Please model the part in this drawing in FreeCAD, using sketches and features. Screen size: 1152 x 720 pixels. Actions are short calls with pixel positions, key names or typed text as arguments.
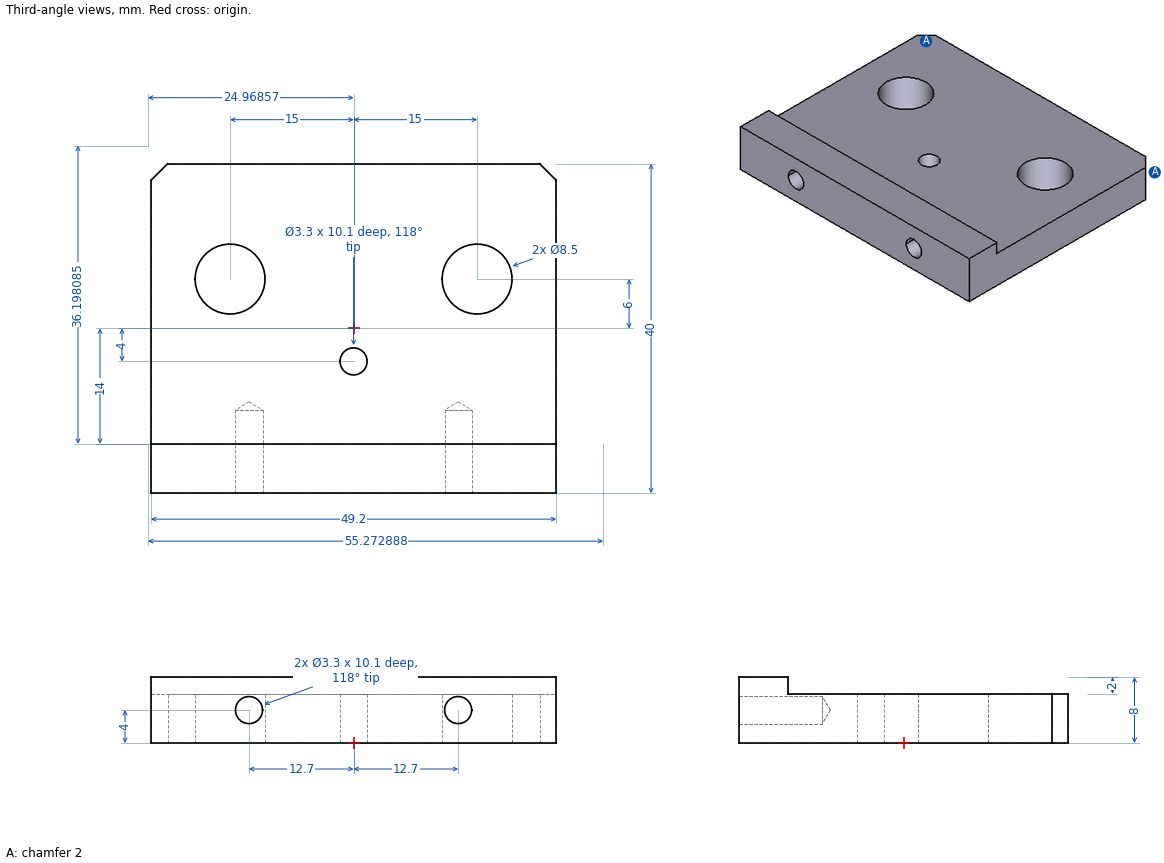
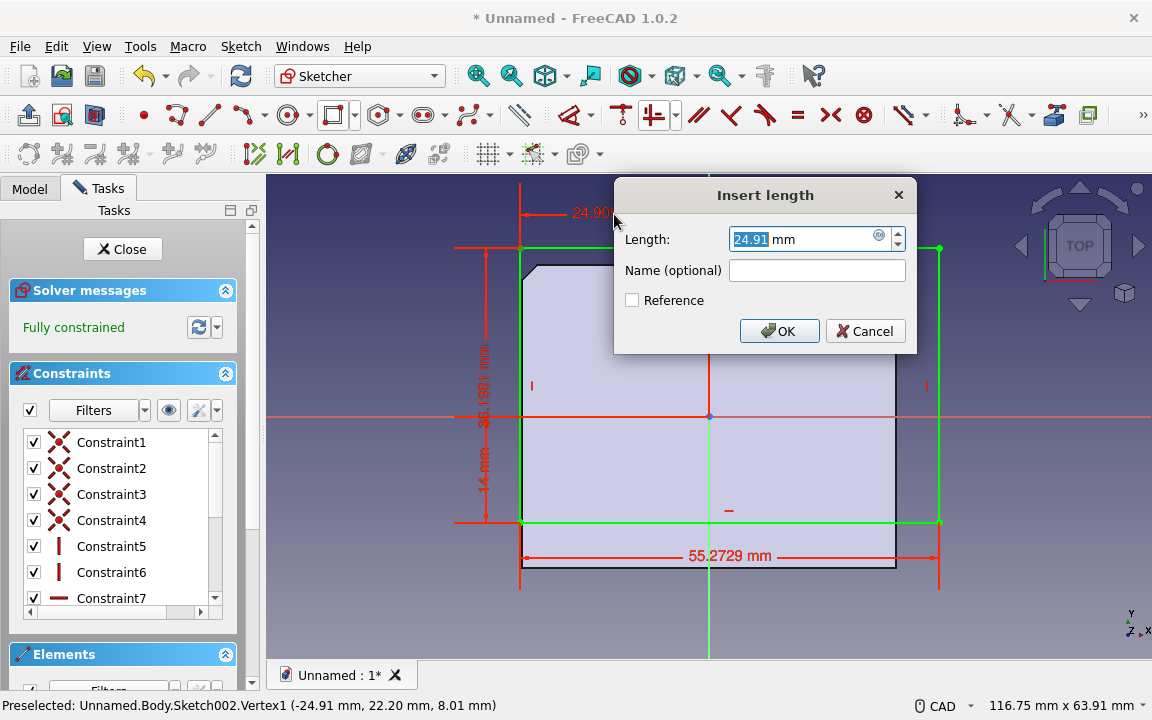
text(24.96857)
key(Return)
key(Escape)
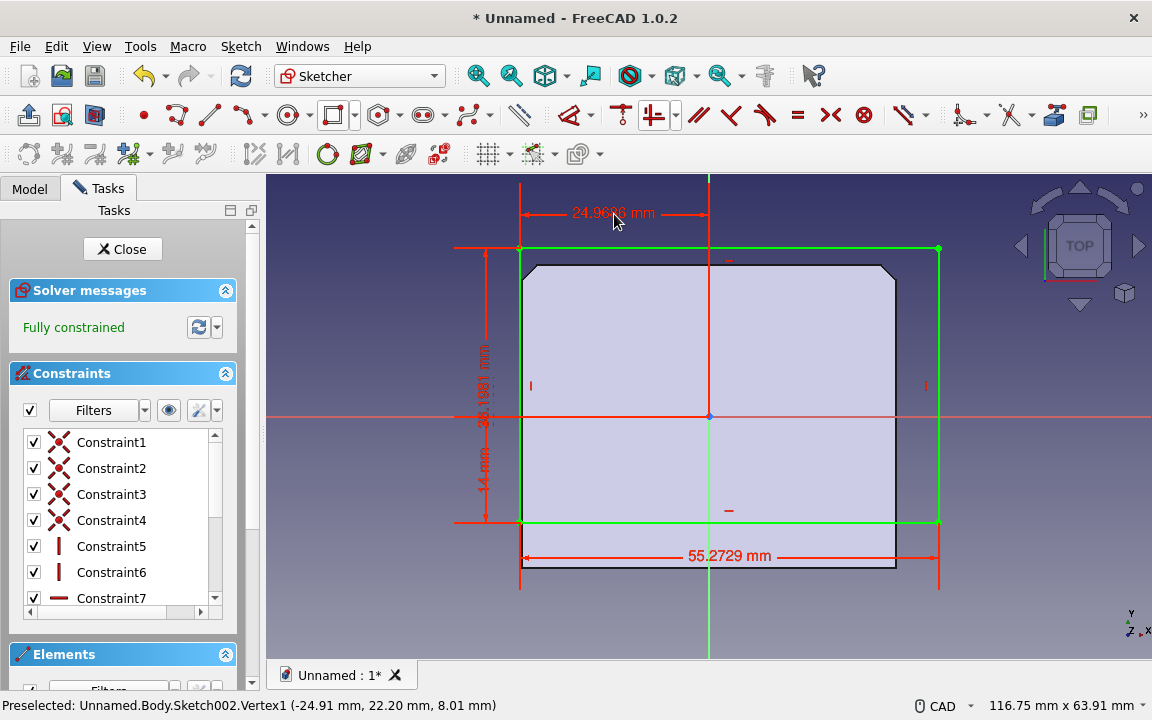
click(123, 249)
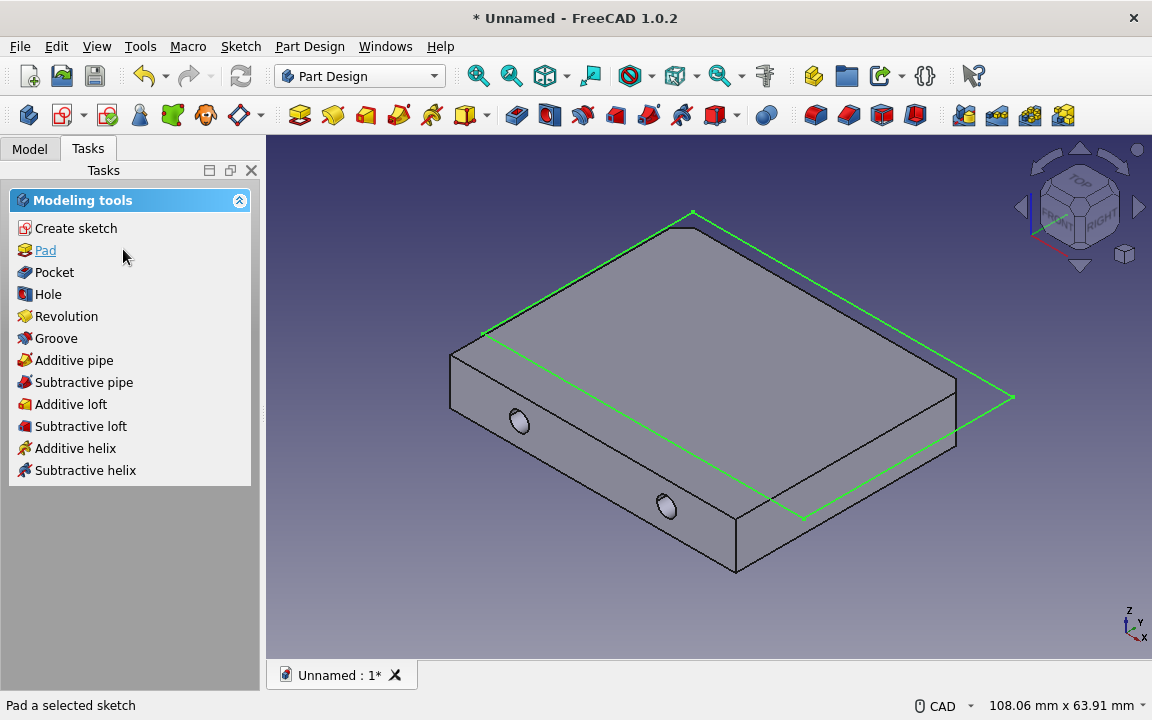
click(517, 116)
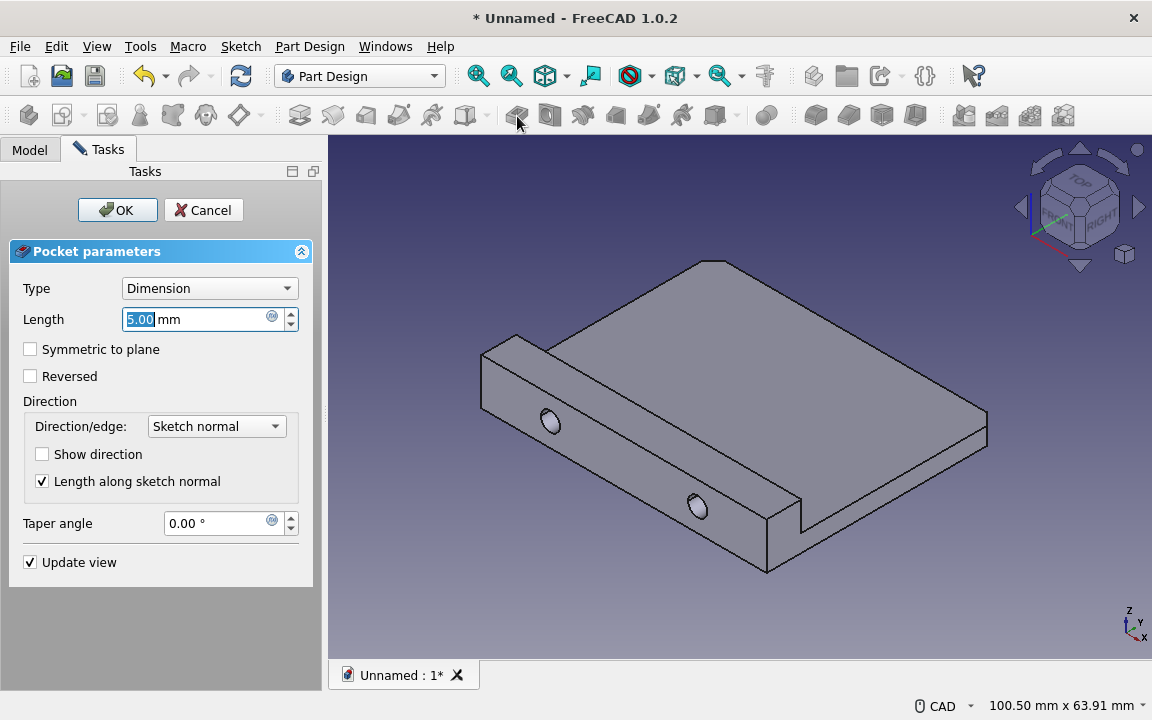
text(2)
key(Tab)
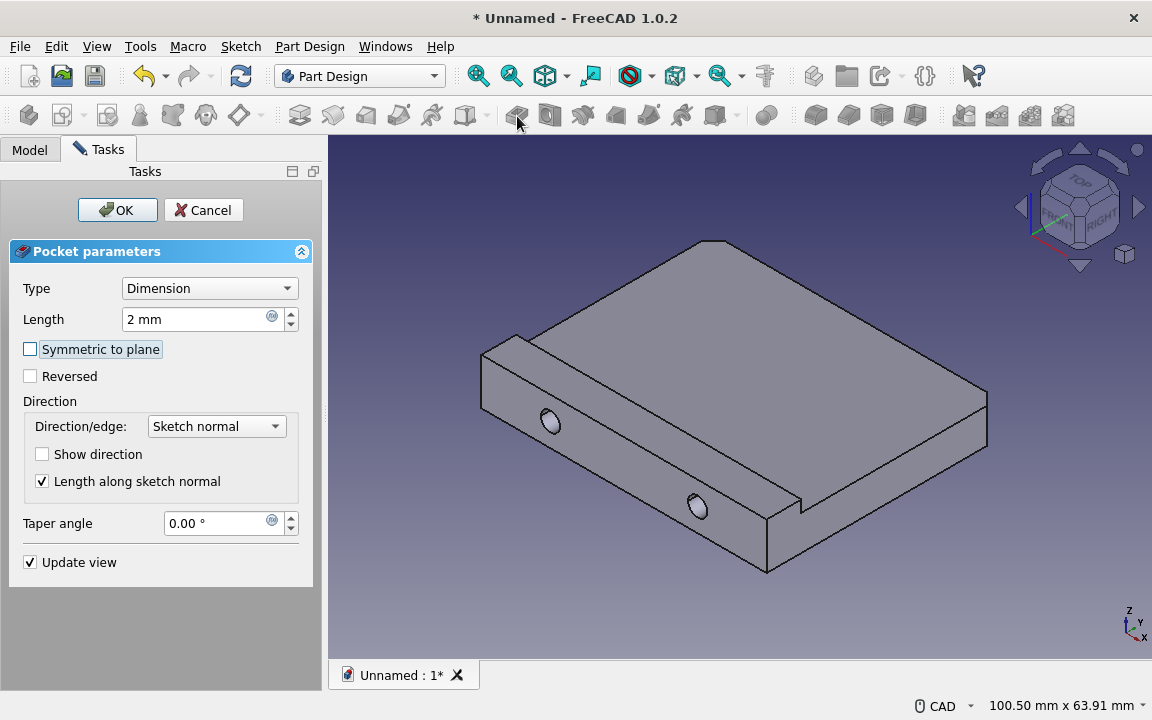
click(118, 210)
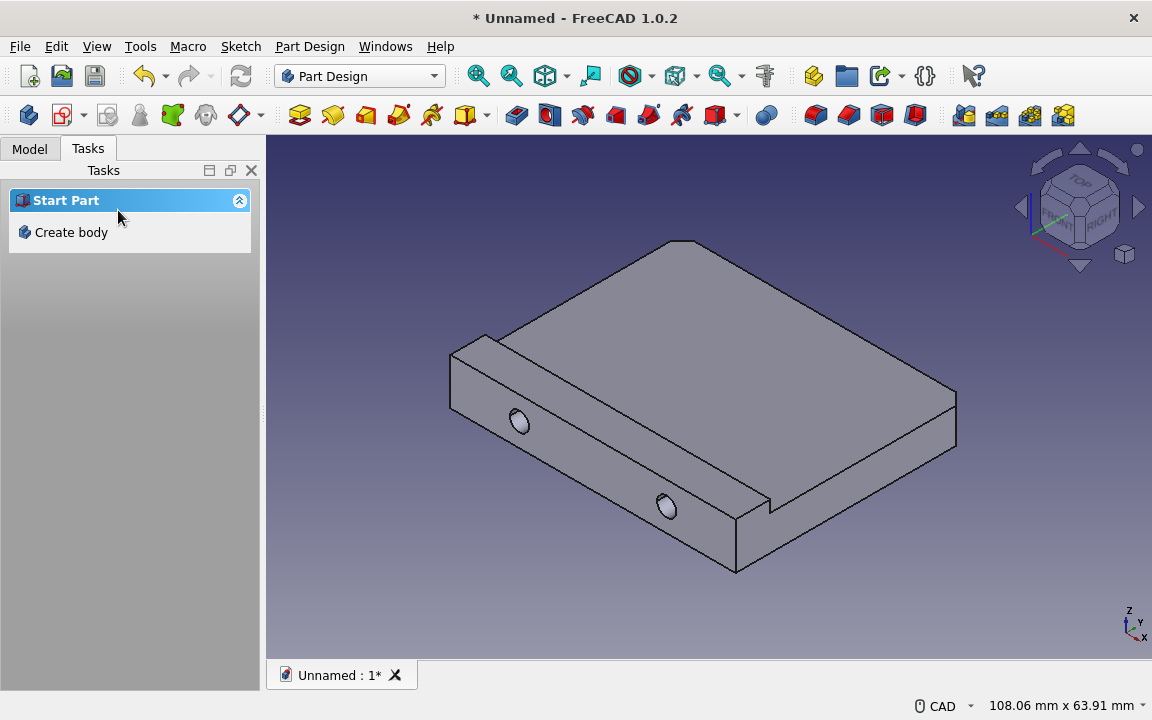
key(5)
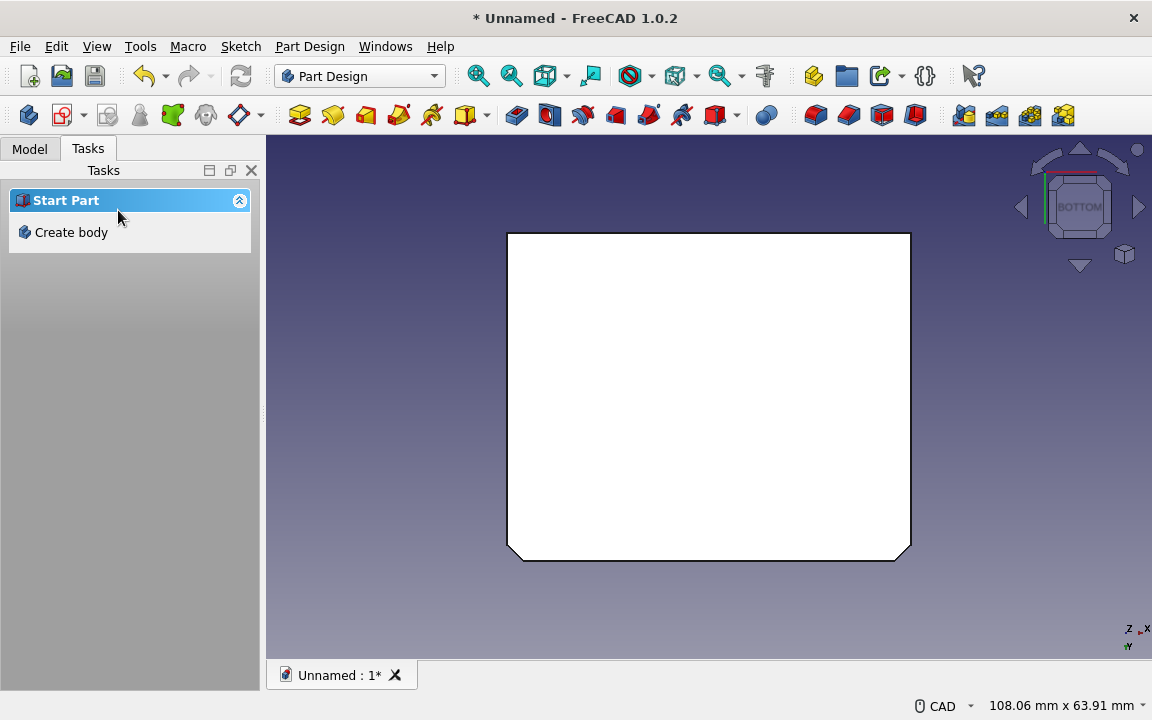
click(709, 396)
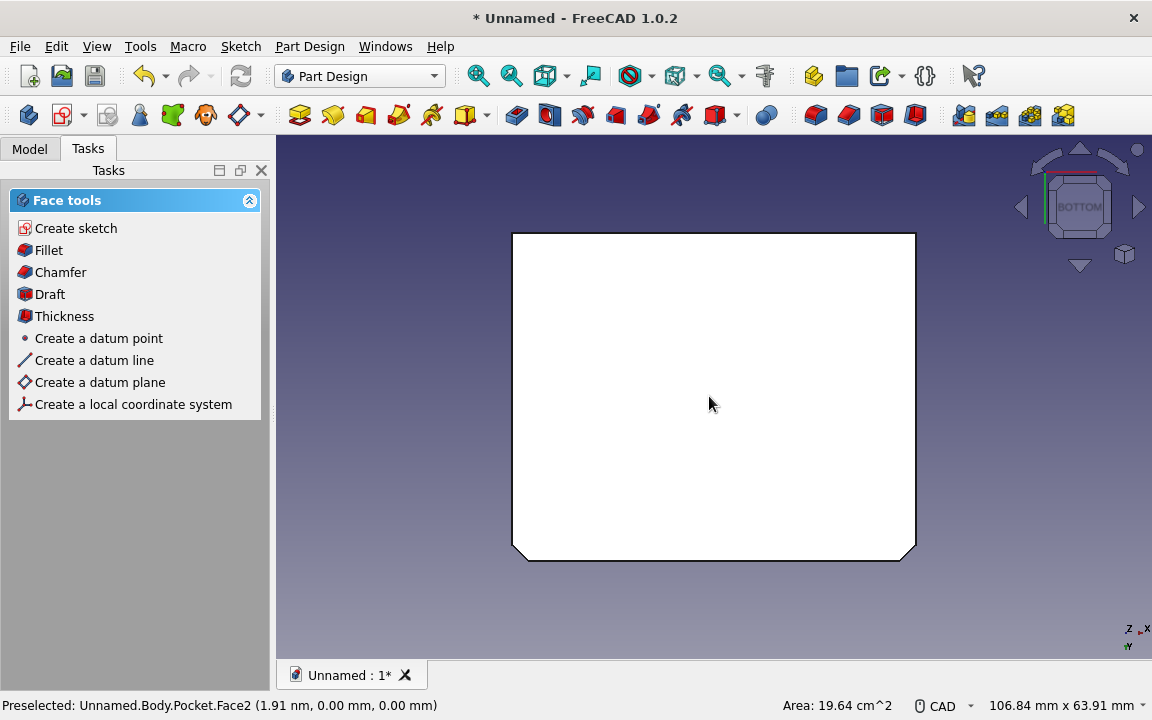
click(62, 116)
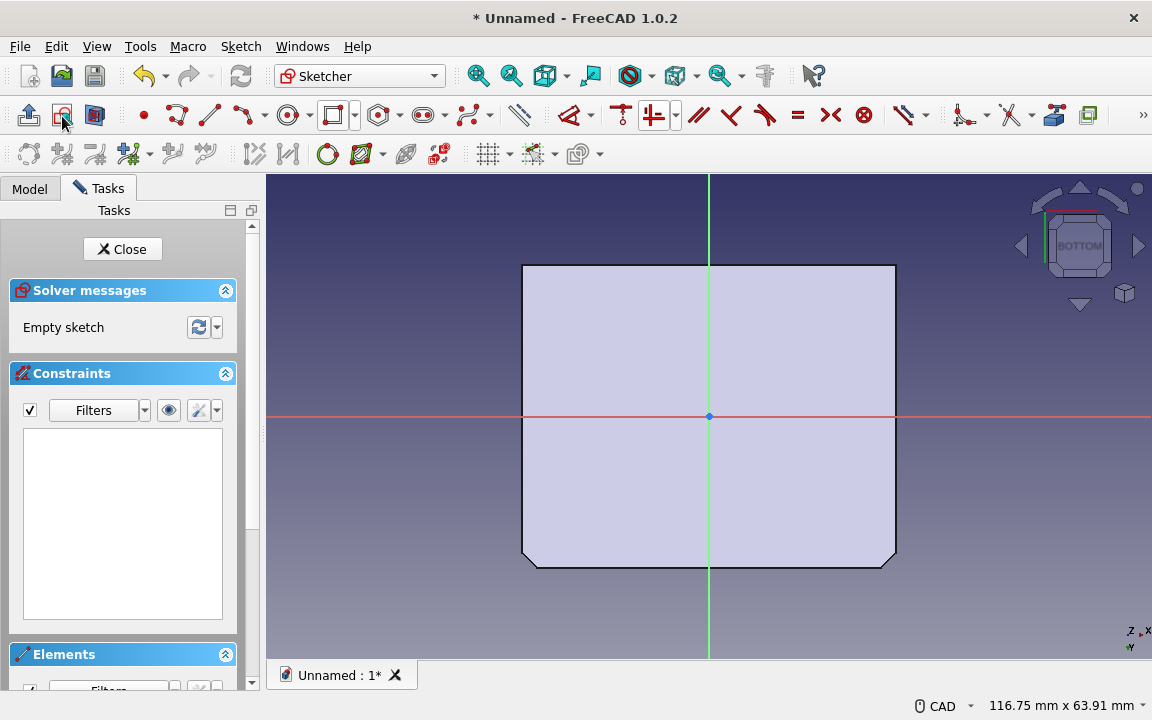
scroll(792, 503, up, 3)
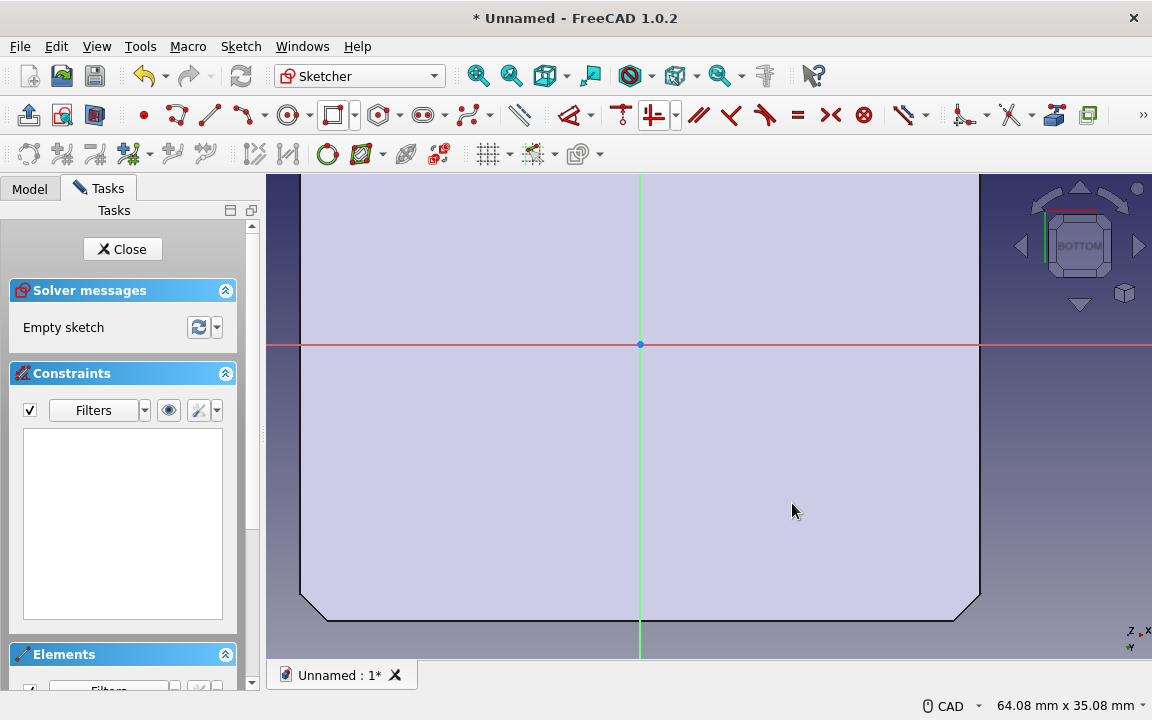
click(288, 116)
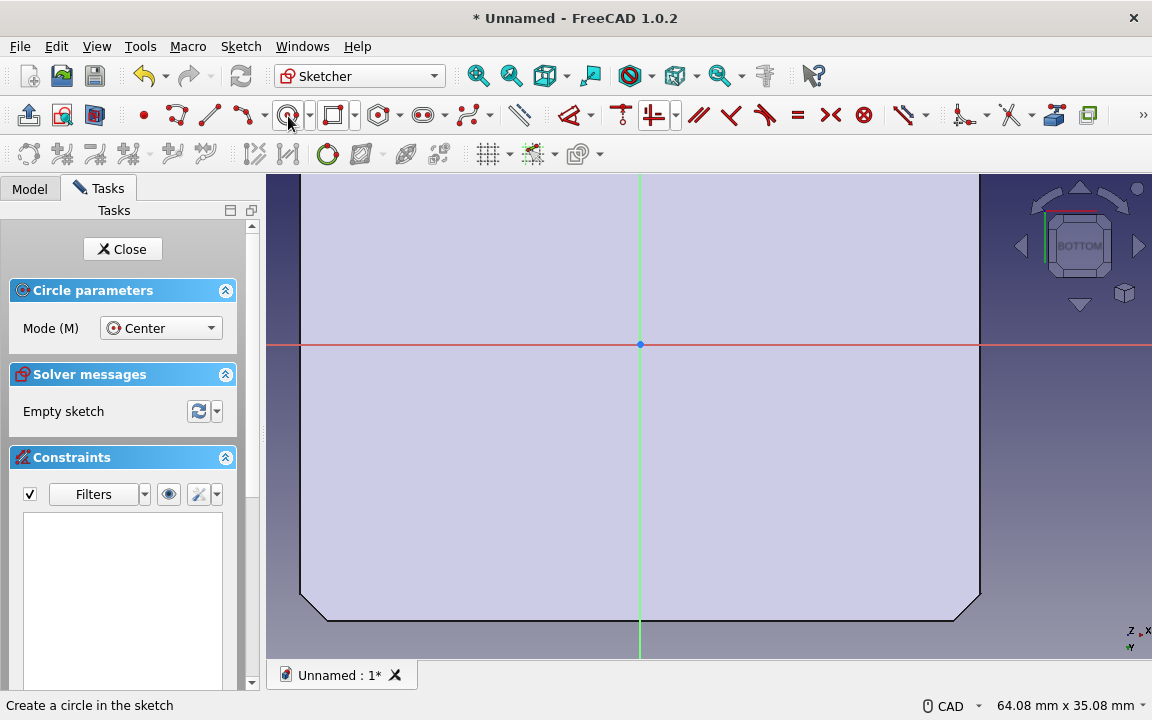
click(848, 428)
click(889, 386)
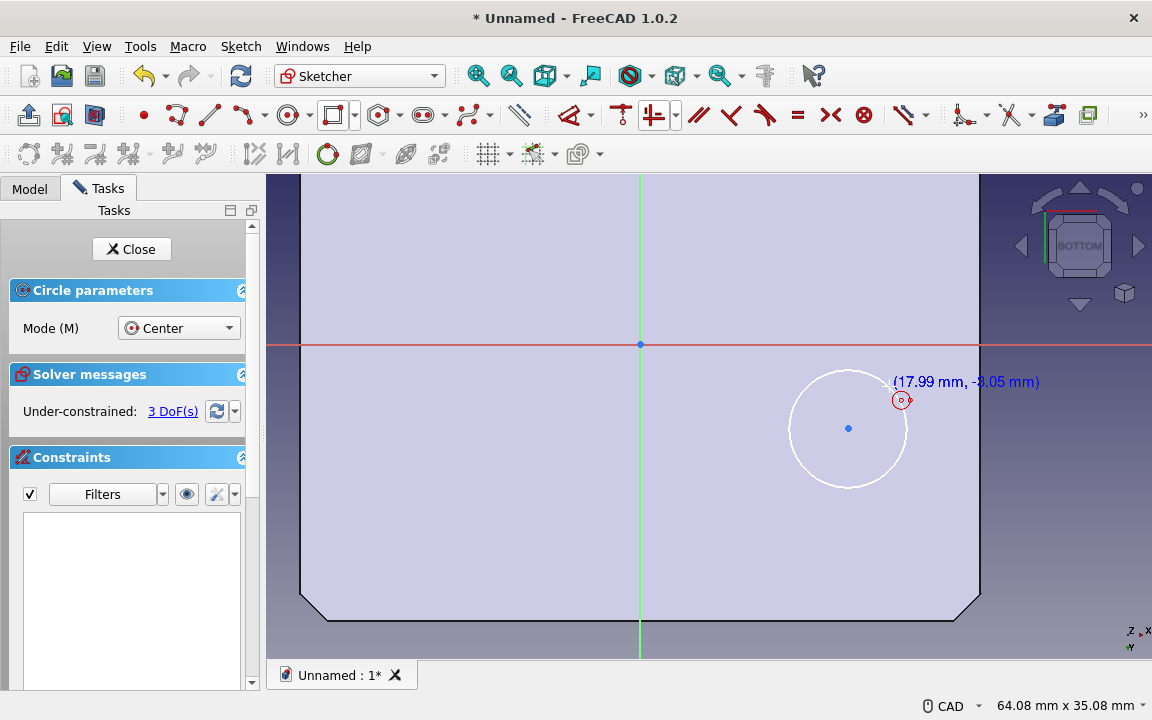
click(433, 428)
click(474, 386)
key(Escape)